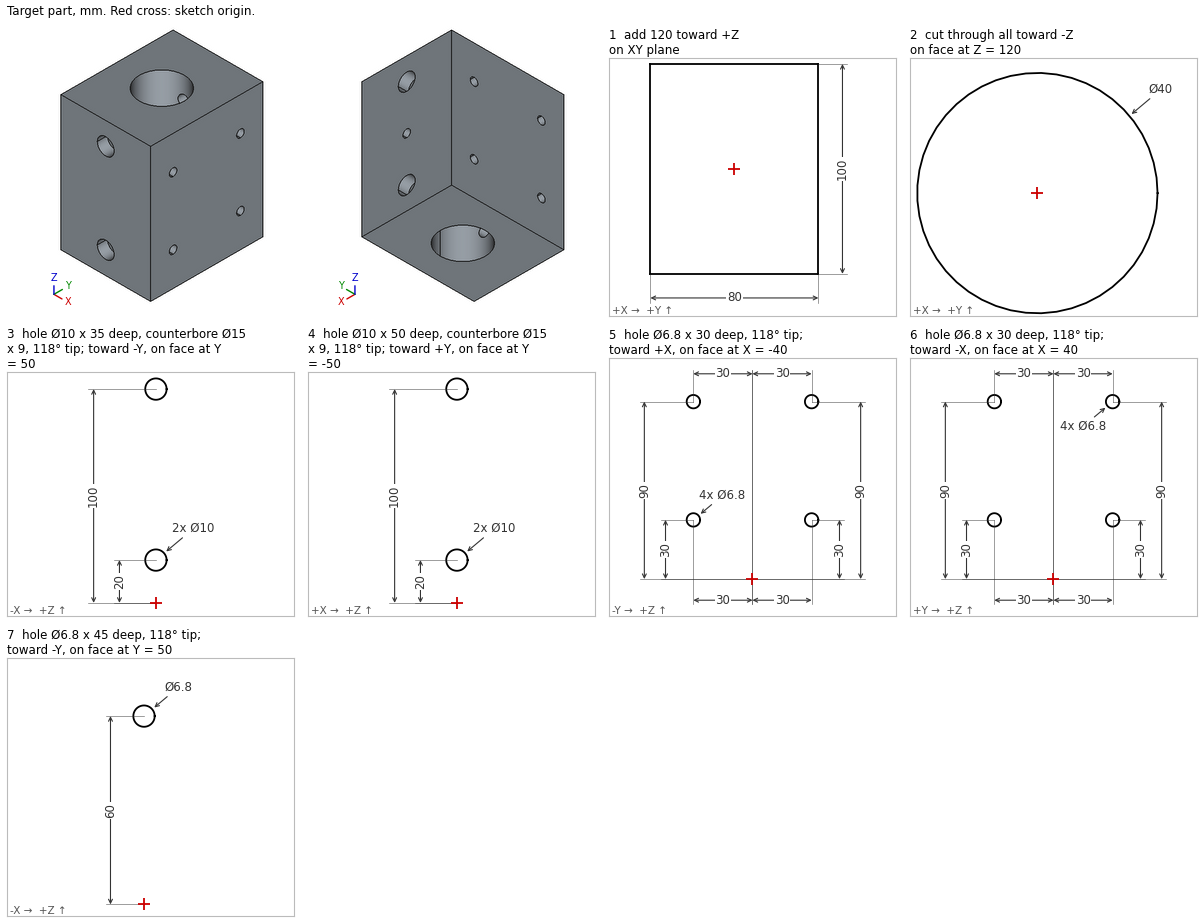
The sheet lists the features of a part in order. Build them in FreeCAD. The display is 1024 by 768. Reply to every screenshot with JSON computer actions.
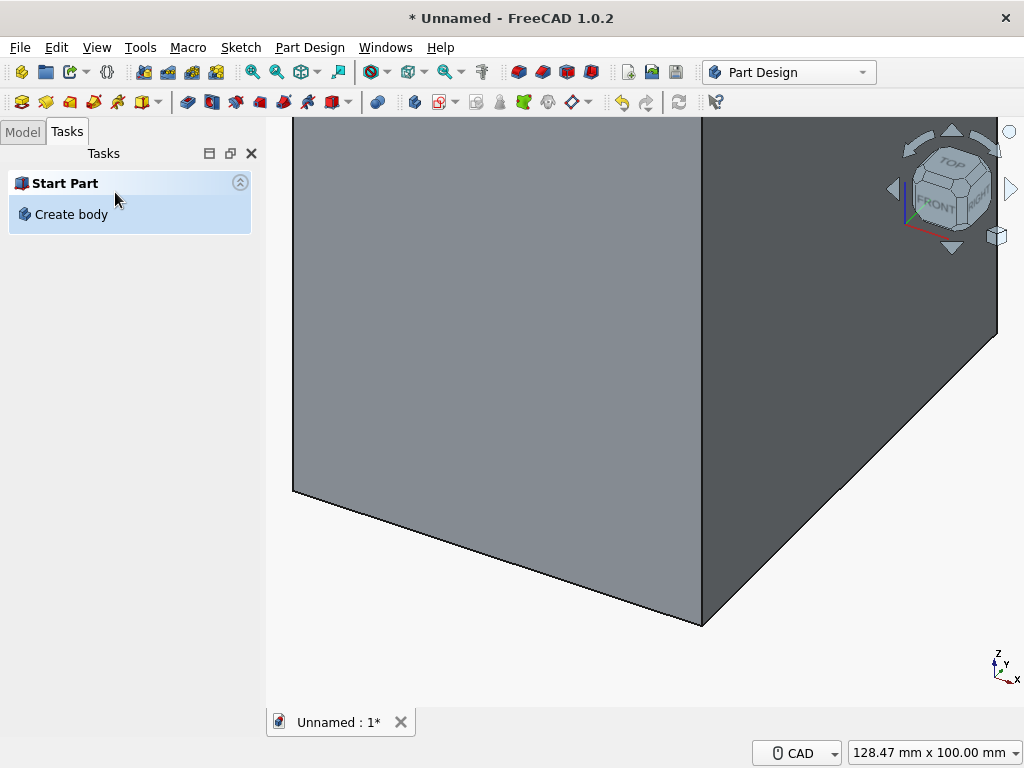
{"action": "left_click", "coordinate": [254, 72]}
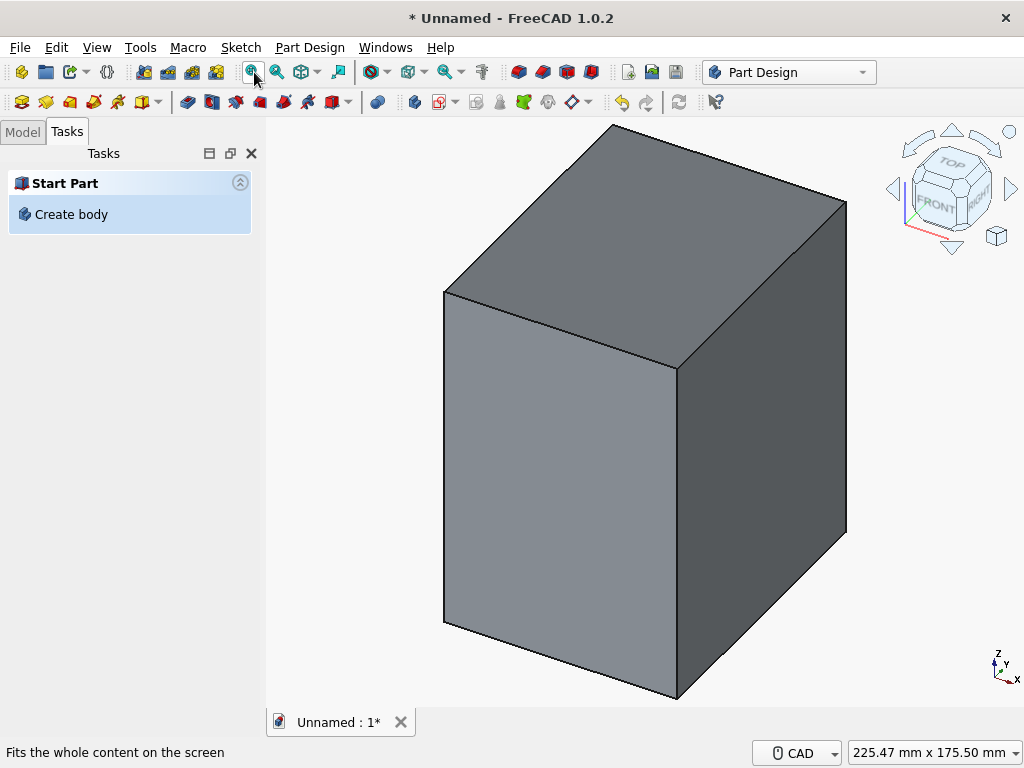
{"action": "left_click", "coordinate": [645, 246]}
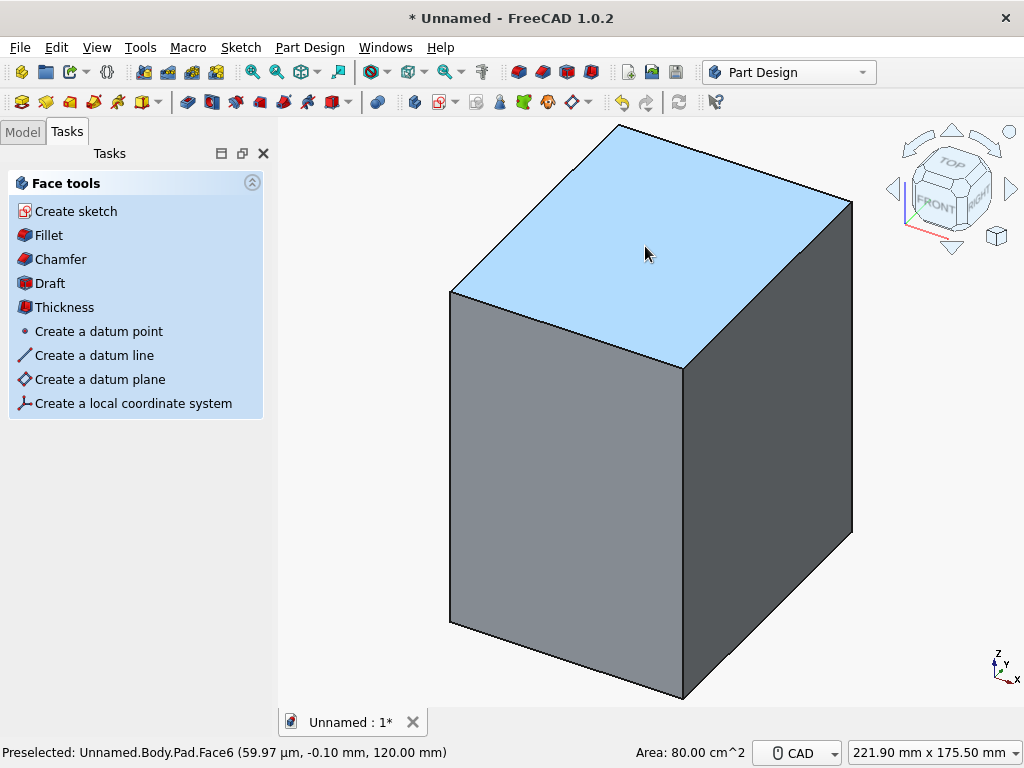
{"action": "left_click", "coordinate": [440, 102]}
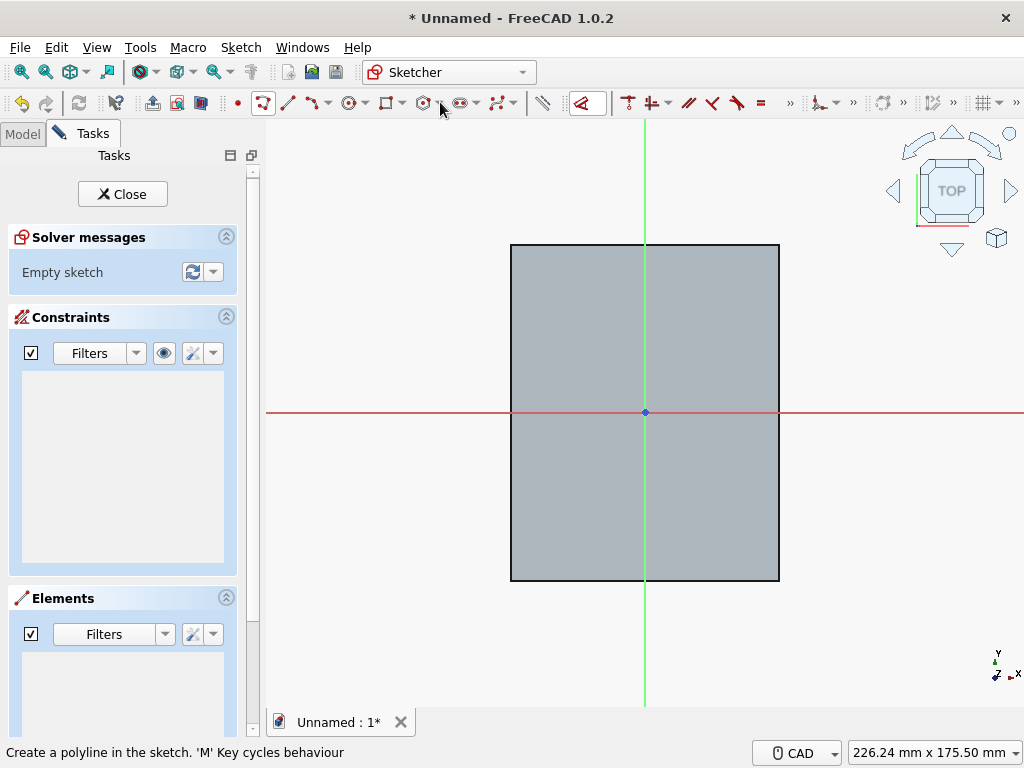
{"action": "scroll", "coordinate": [685, 413], "scroll_direction": "up", "scroll_amount": 5}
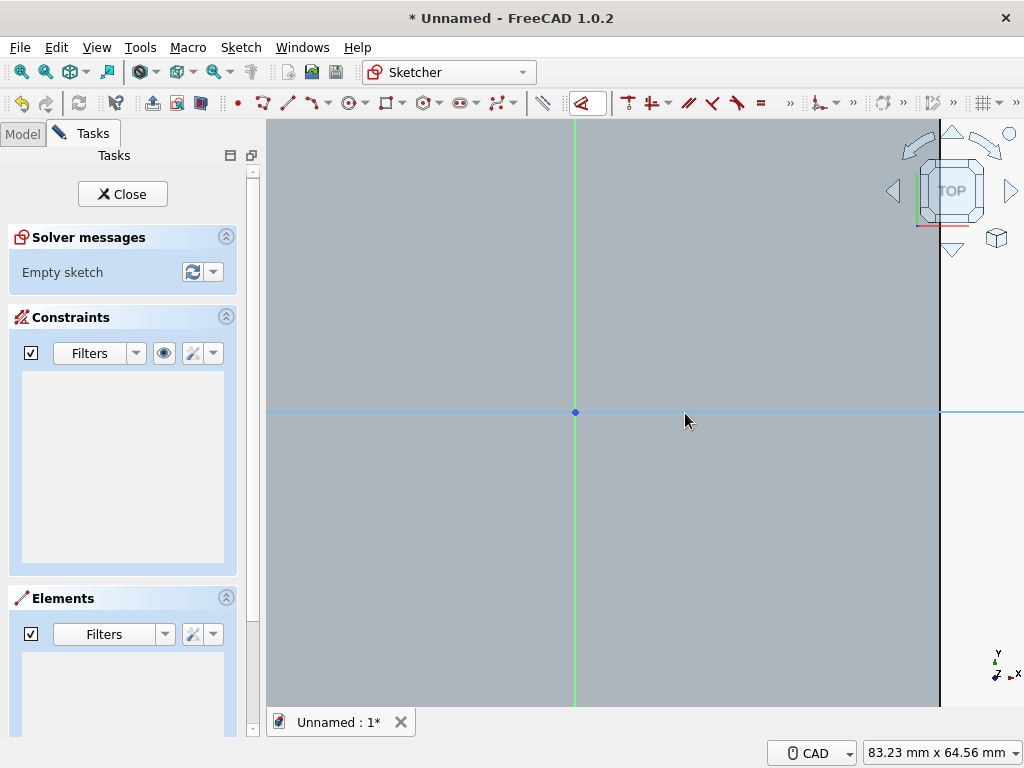
{"action": "left_click", "coordinate": [350, 104]}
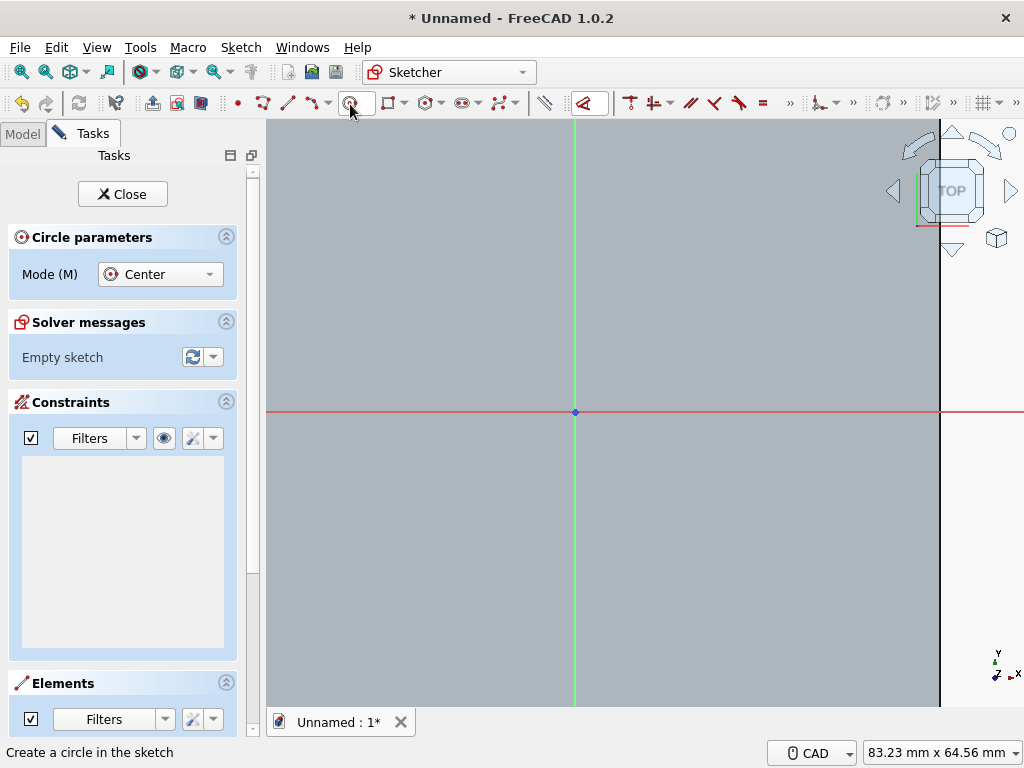
{"action": "left_click", "coordinate": [575, 412]}
{"action": "mouse_move", "coordinate": [704, 283]}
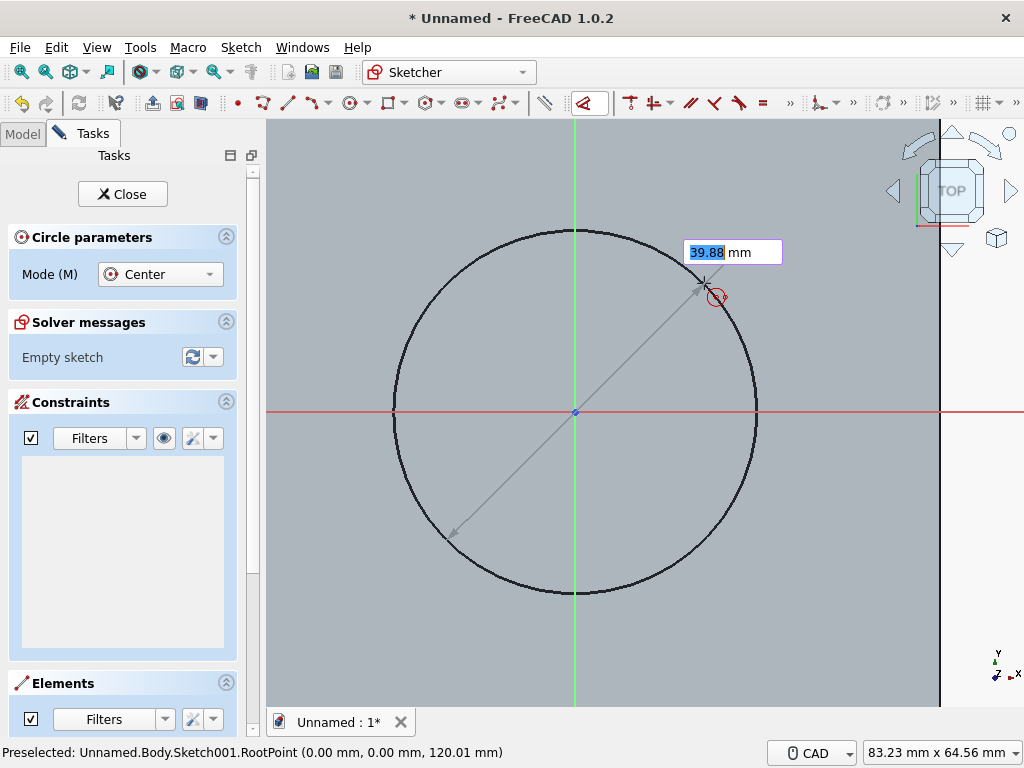
{"action": "type", "text": "40"}
{"action": "key", "text": "Return"}
{"action": "key", "text": "Escape"}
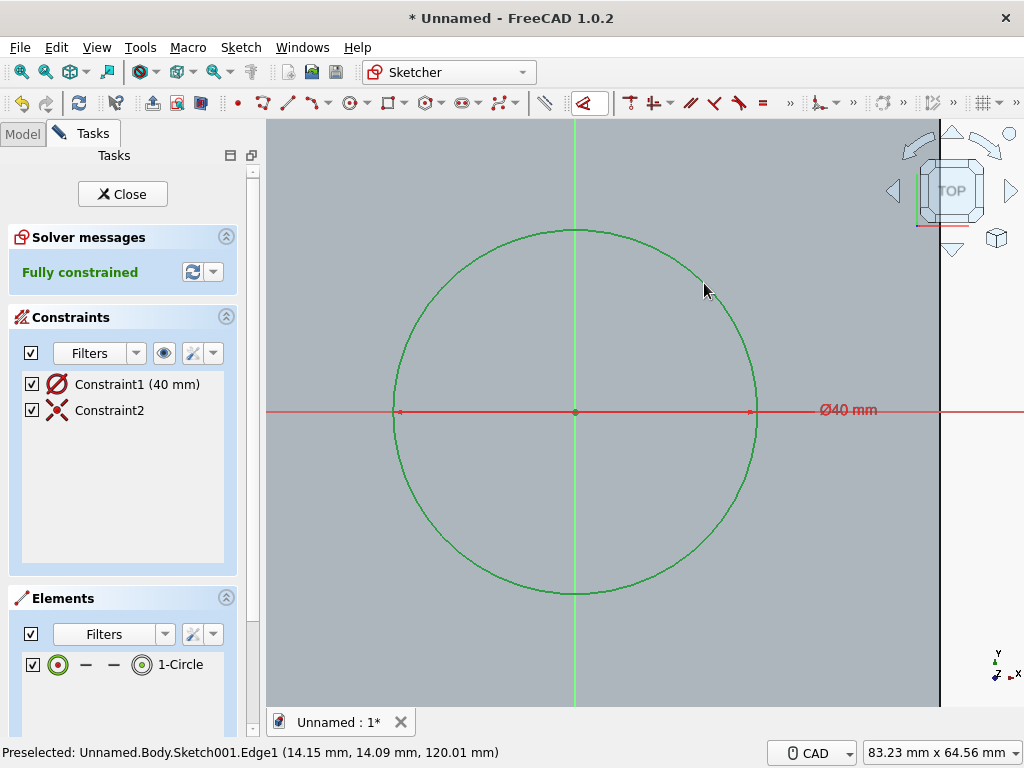
{"action": "left_click", "coordinate": [123, 194]}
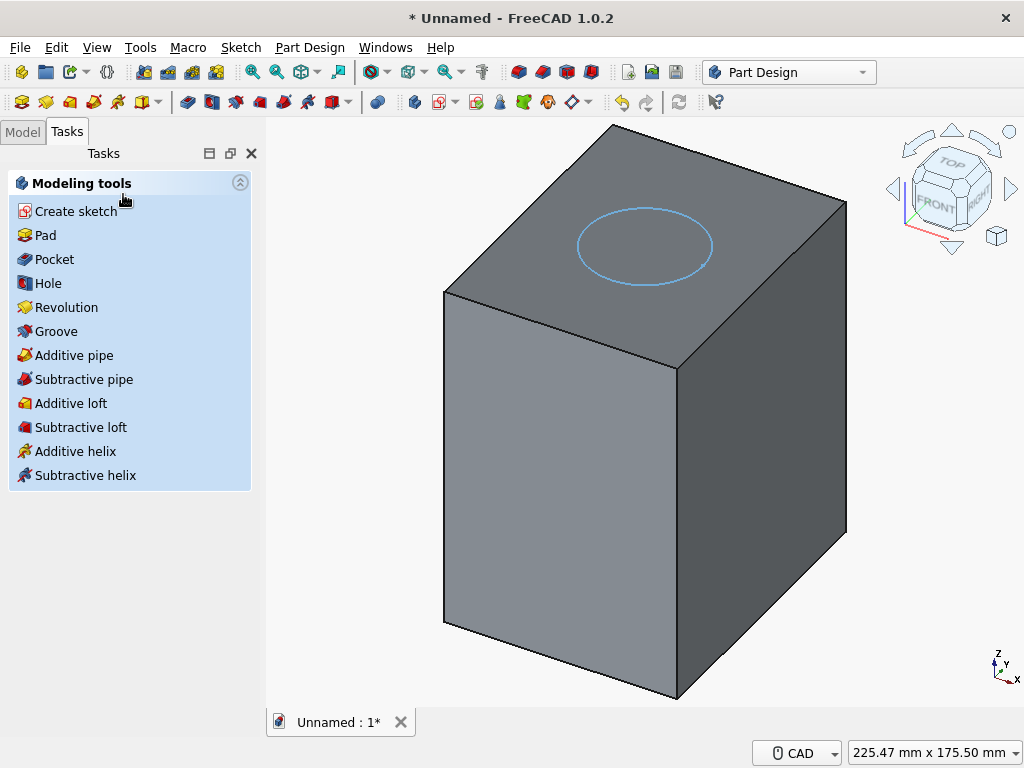
{"action": "left_click", "coordinate": [188, 102]}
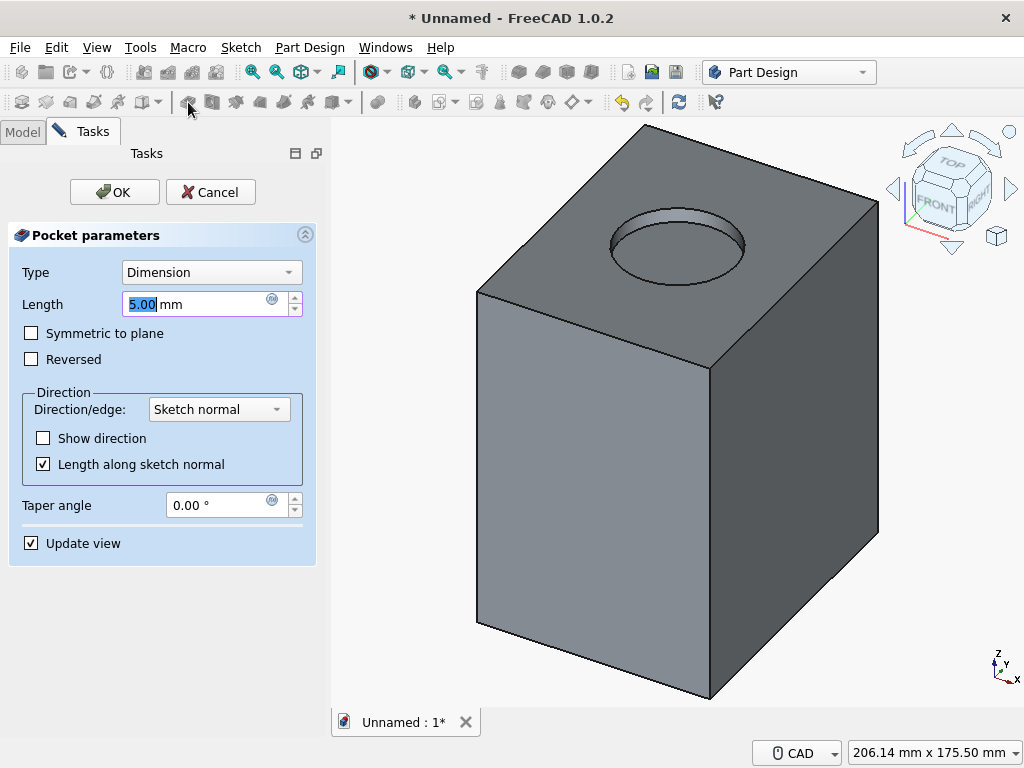
{"action": "left_click", "coordinate": [212, 272]}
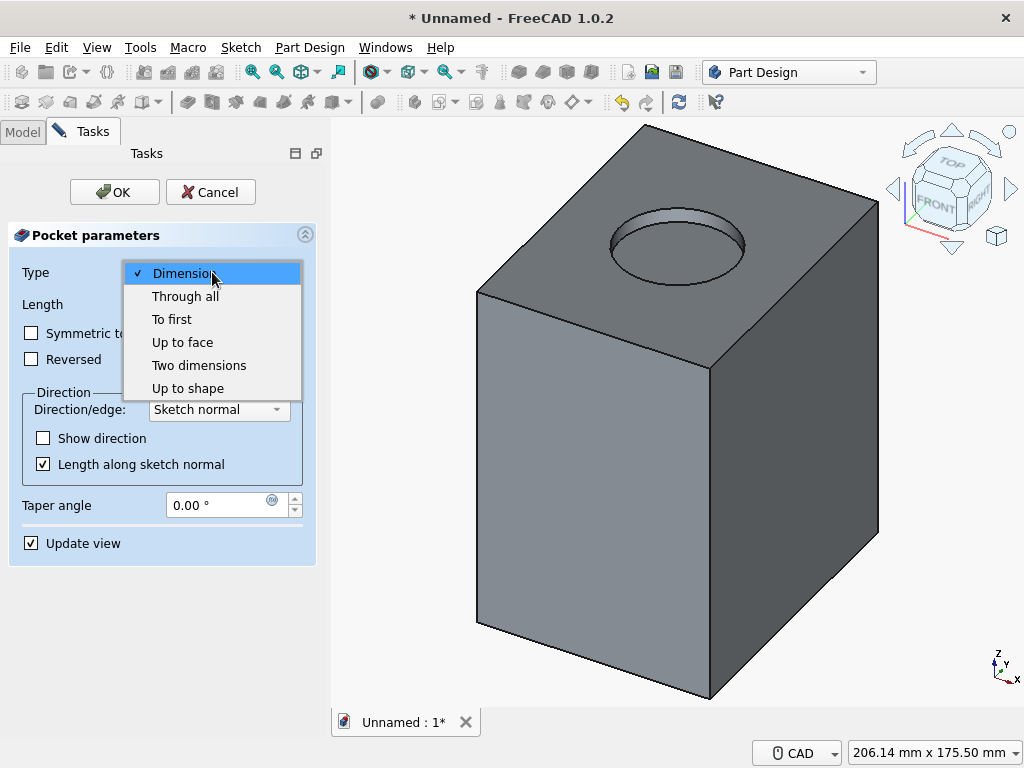
{"action": "left_click", "coordinate": [212, 296]}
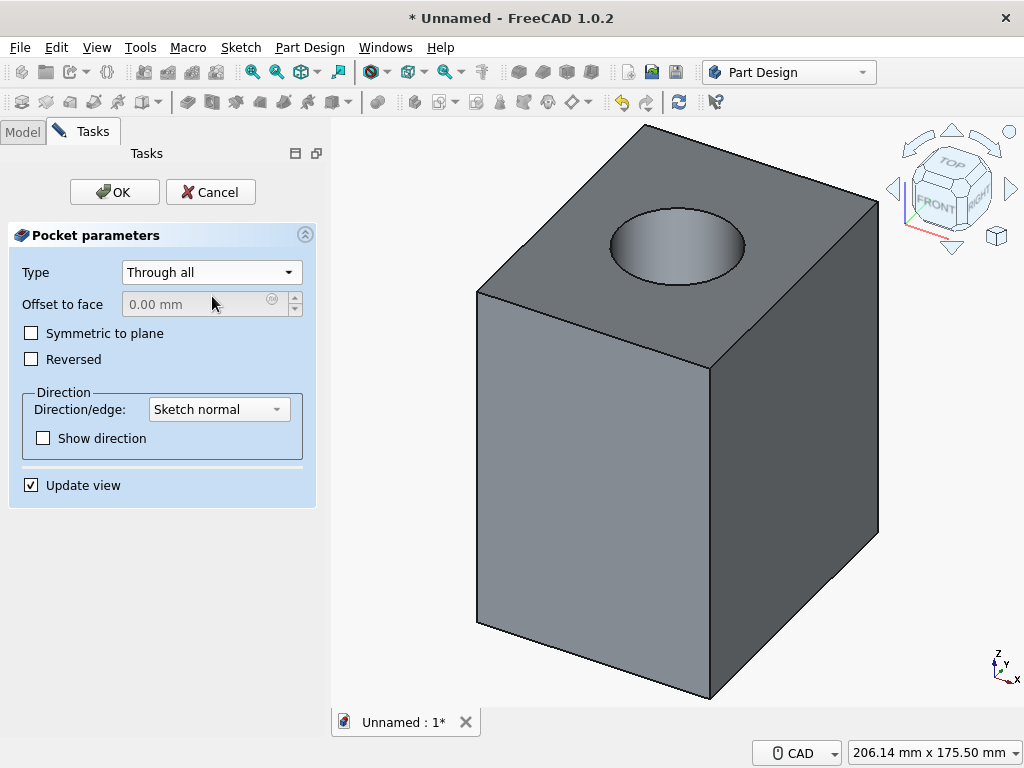
{"action": "left_click", "coordinate": [115, 192]}